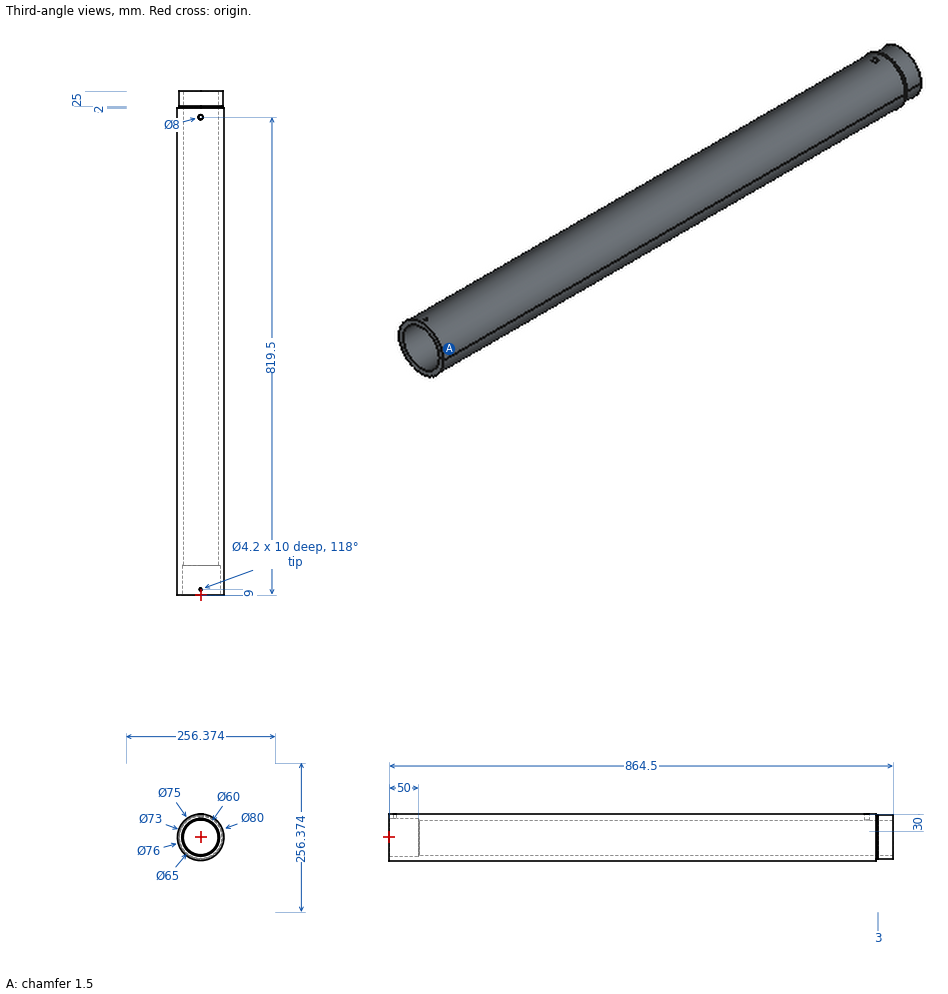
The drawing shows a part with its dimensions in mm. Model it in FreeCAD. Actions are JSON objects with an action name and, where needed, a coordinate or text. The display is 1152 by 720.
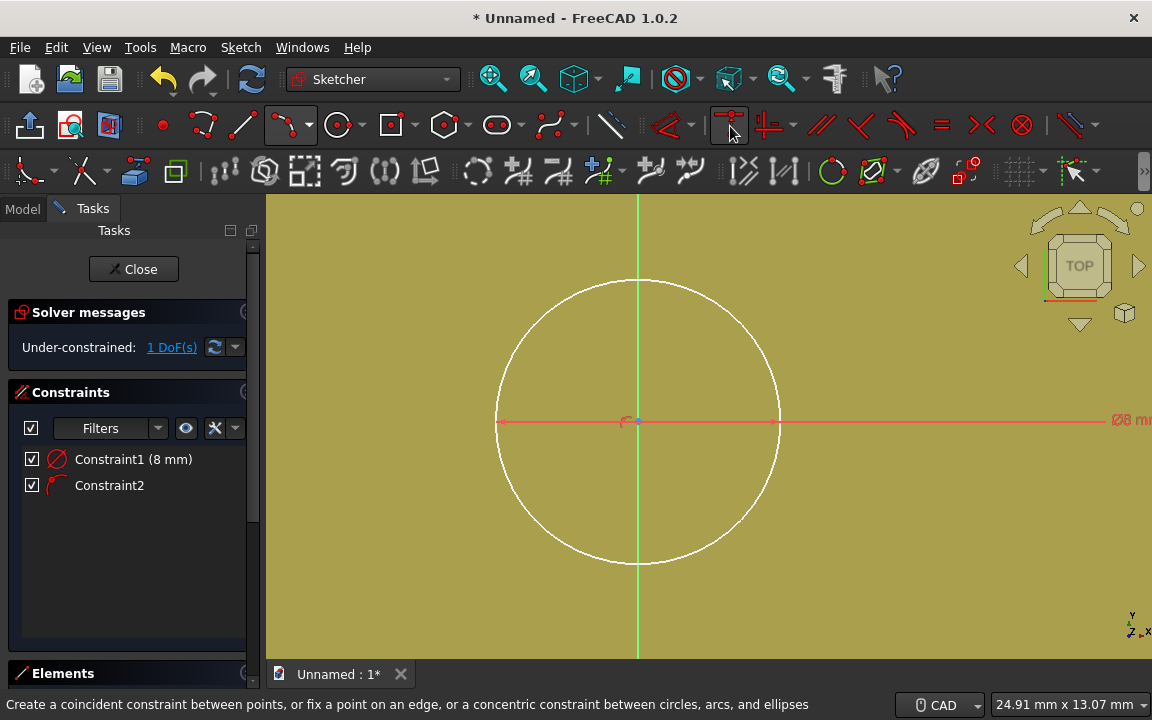
{"action": "left_click", "coordinate": [666, 126]}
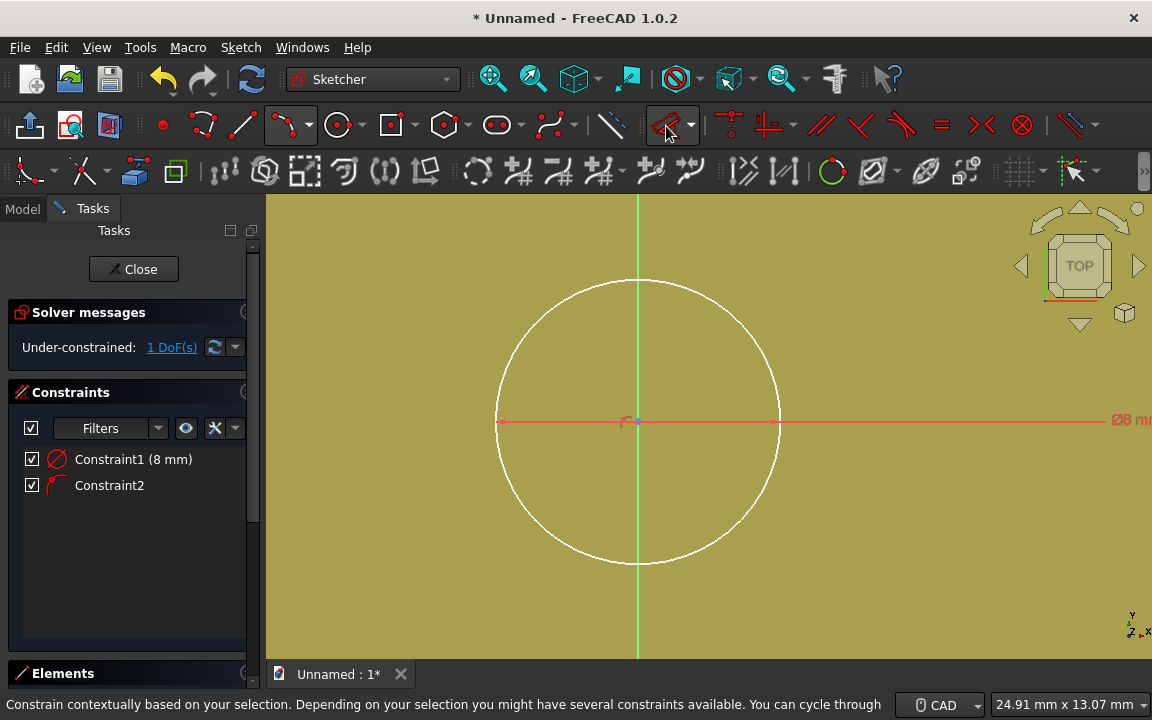
{"action": "left_click", "coordinate": [638, 422]}
{"action": "left_click", "coordinate": [672, 526]}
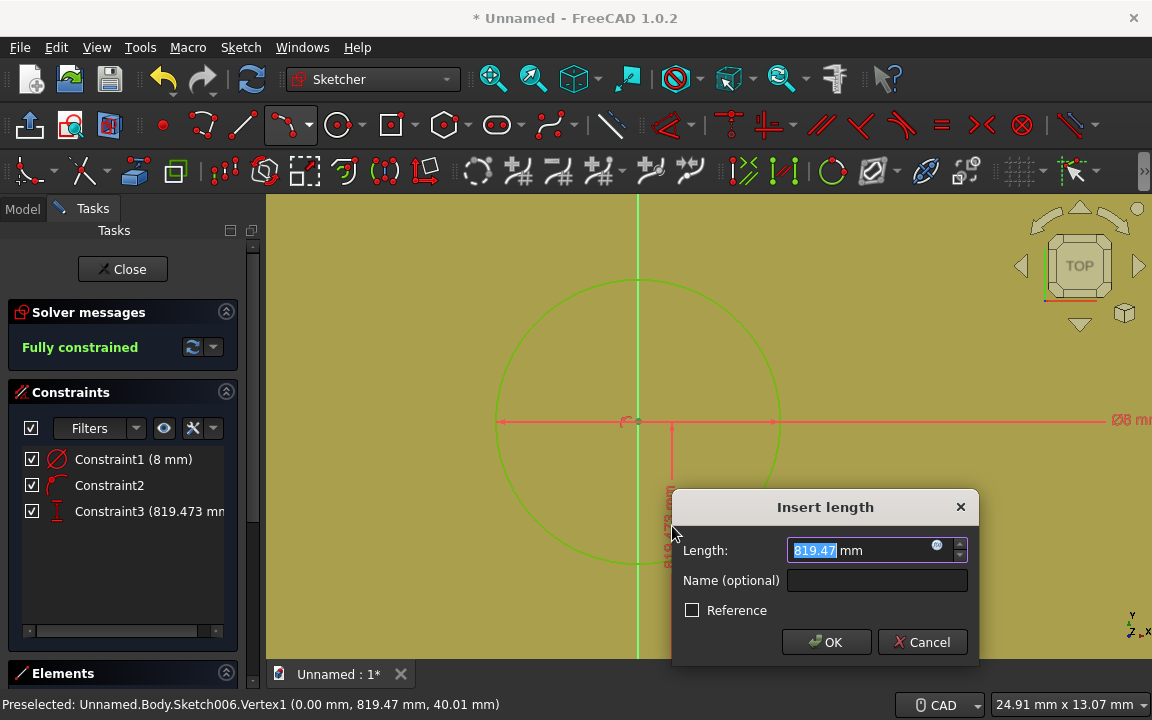
{"action": "type", "text": "819.5"}
{"action": "key", "text": "Return"}
{"action": "key", "text": "Escape"}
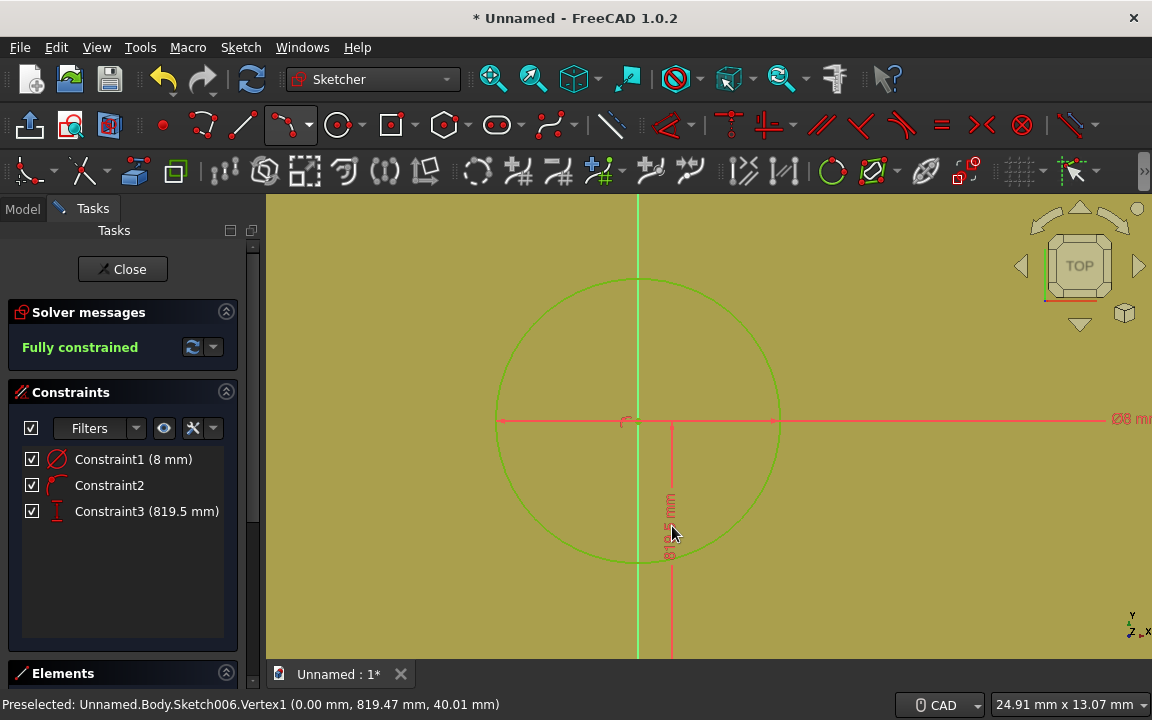
{"action": "left_click", "coordinate": [123, 269]}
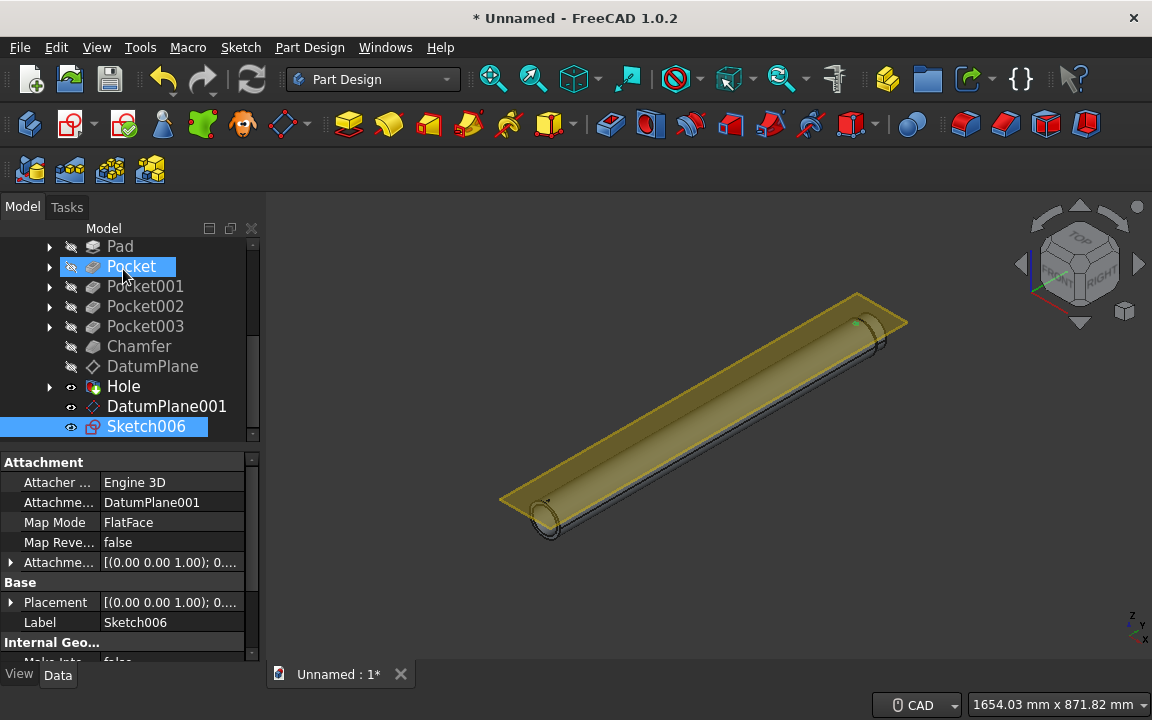
{"action": "left_click", "coordinate": [612, 124]}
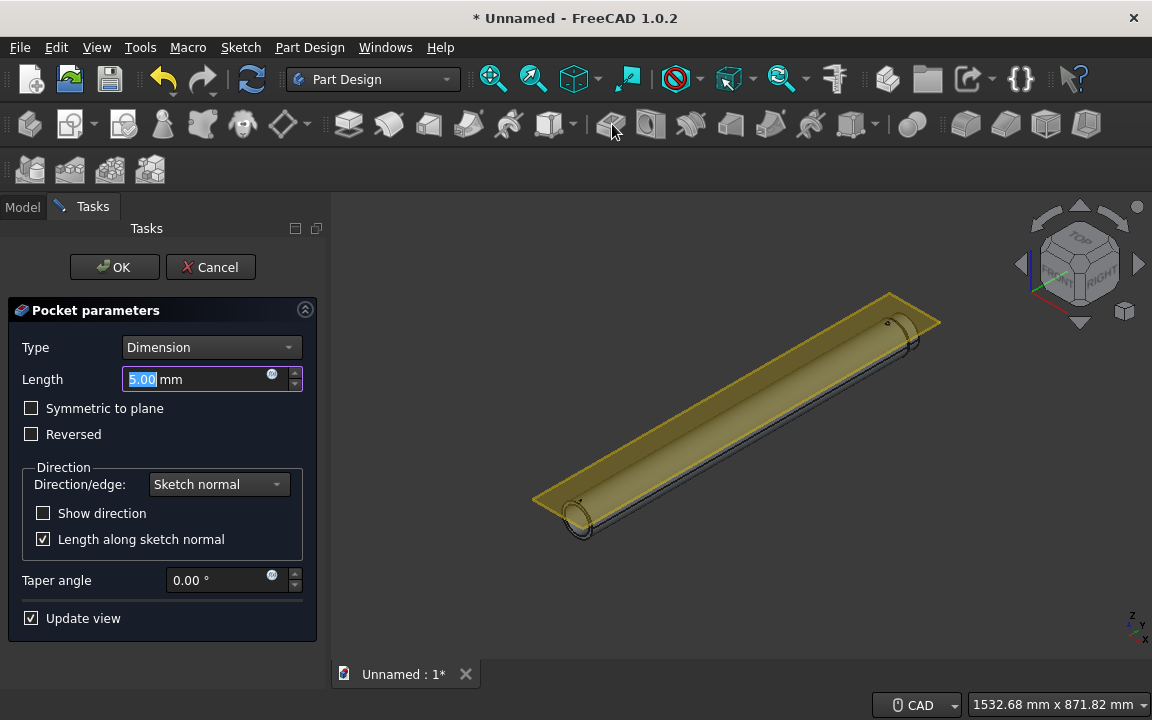
{"action": "type", "text": "30"}
{"action": "key", "text": "Tab"}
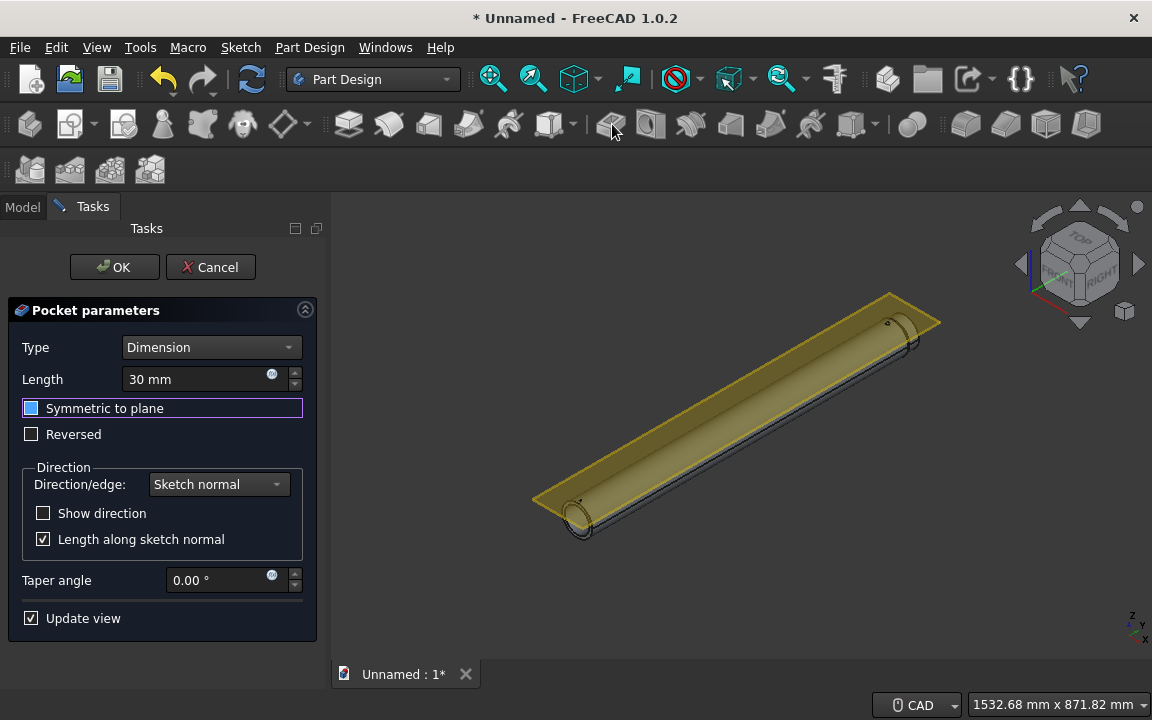
{"action": "left_click", "coordinate": [115, 267]}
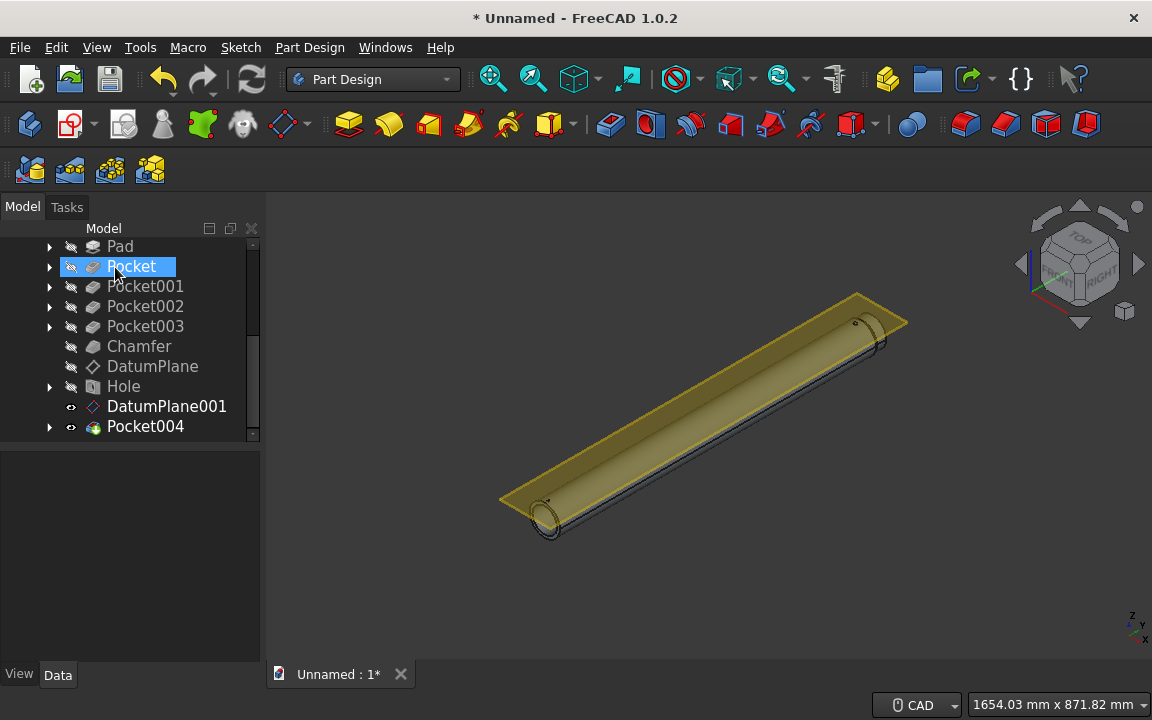
{"action": "left_click", "coordinate": [116, 407]}
{"action": "key", "text": "space"}